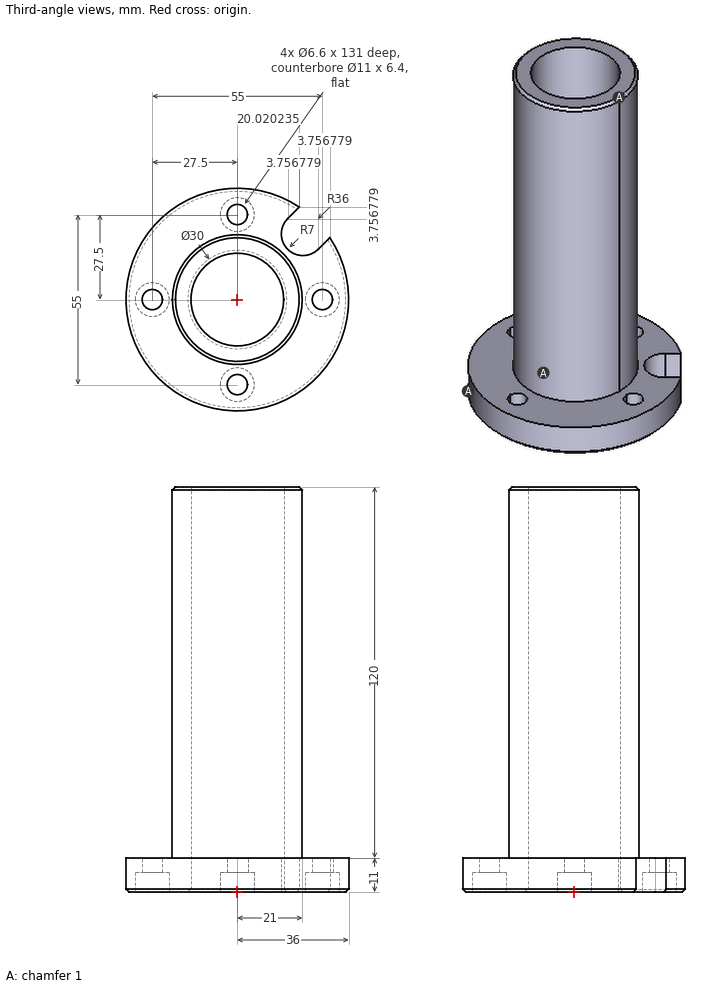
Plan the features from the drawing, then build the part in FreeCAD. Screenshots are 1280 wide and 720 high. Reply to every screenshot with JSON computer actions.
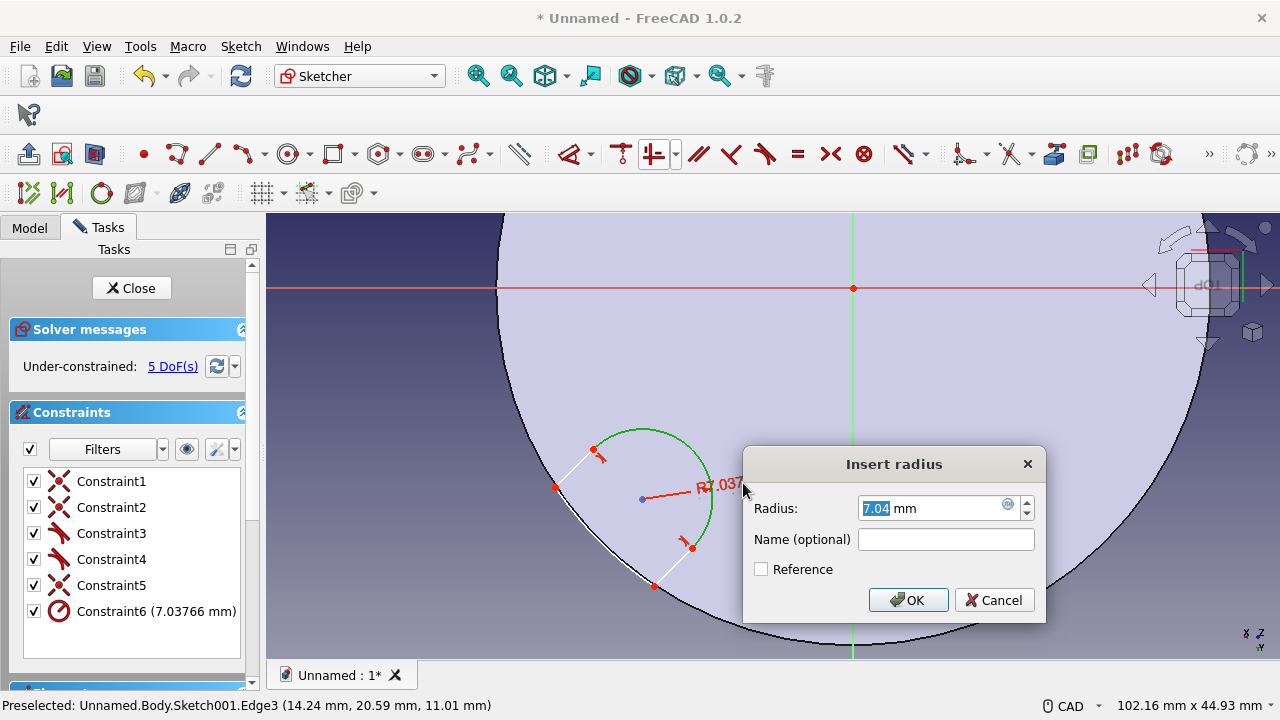
{"action": "type", "text": "7"}
{"action": "key", "text": "Return"}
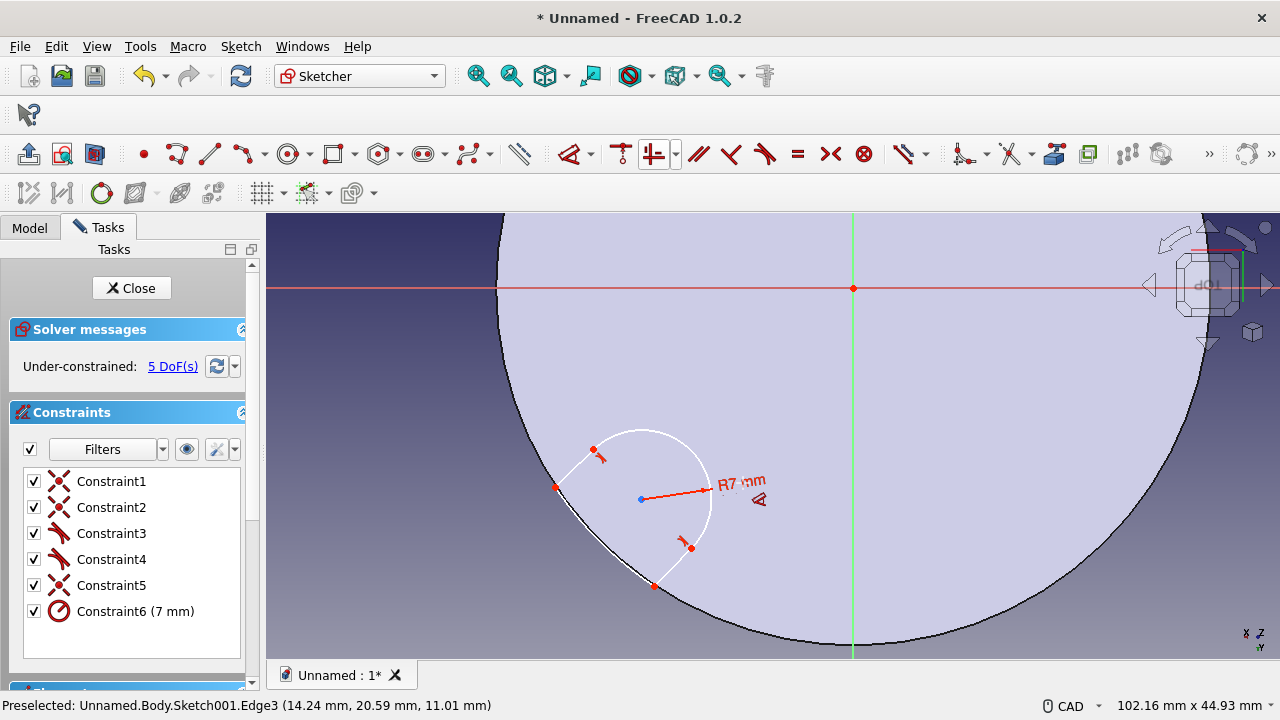
{"action": "left_click", "coordinate": [581, 521]}
{"action": "left_click", "coordinate": [557, 542]}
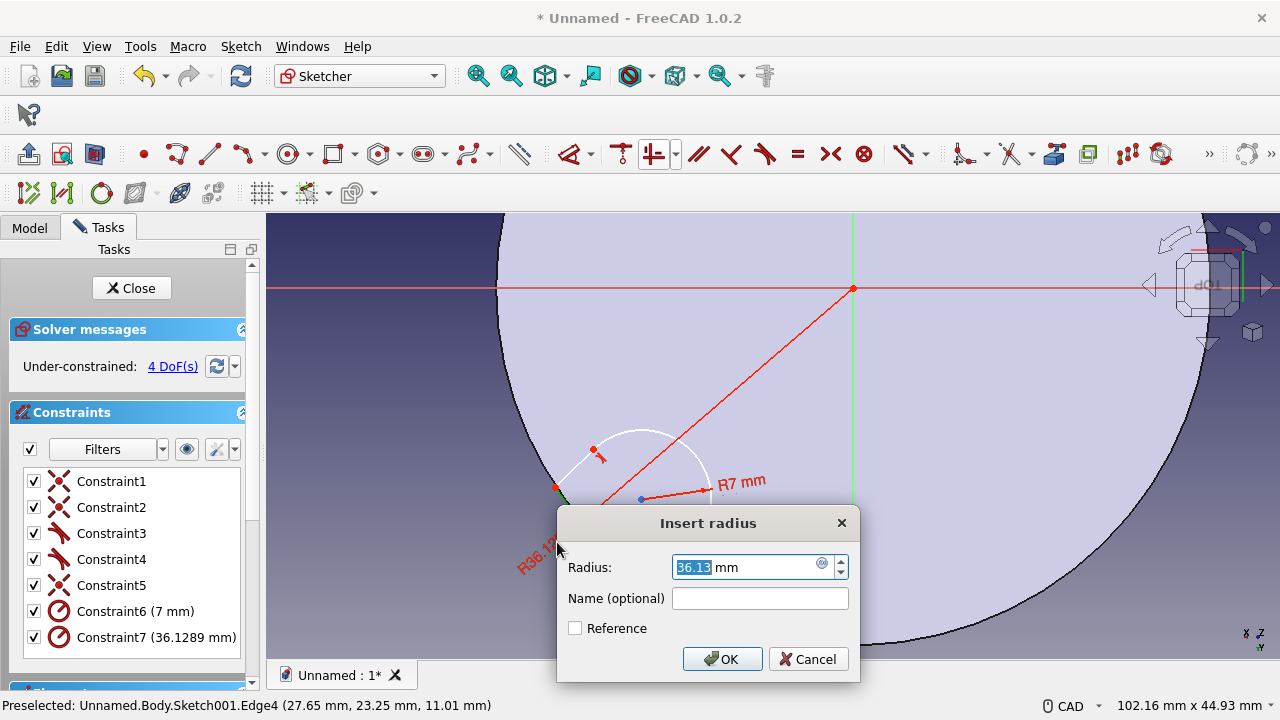
{"action": "type", "text": "36"}
{"action": "key", "text": "Return"}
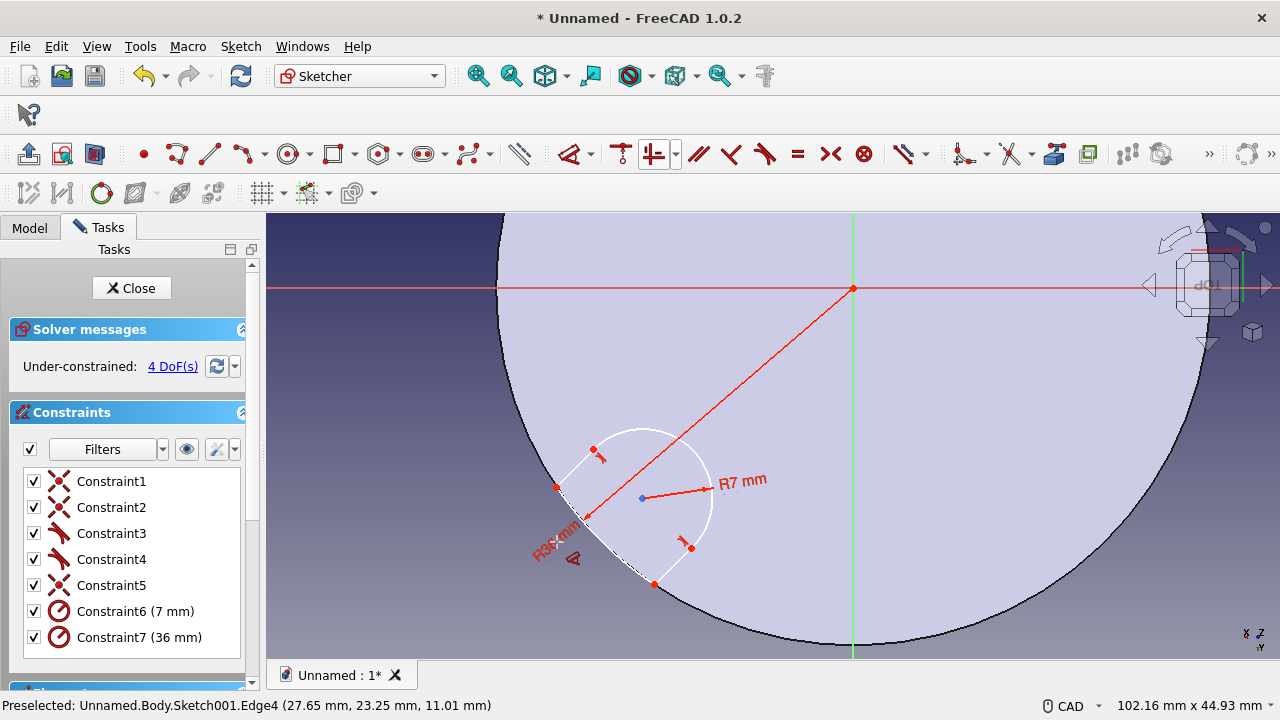
{"action": "left_click", "coordinate": [665, 574]}
{"action": "left_click", "coordinate": [673, 619]}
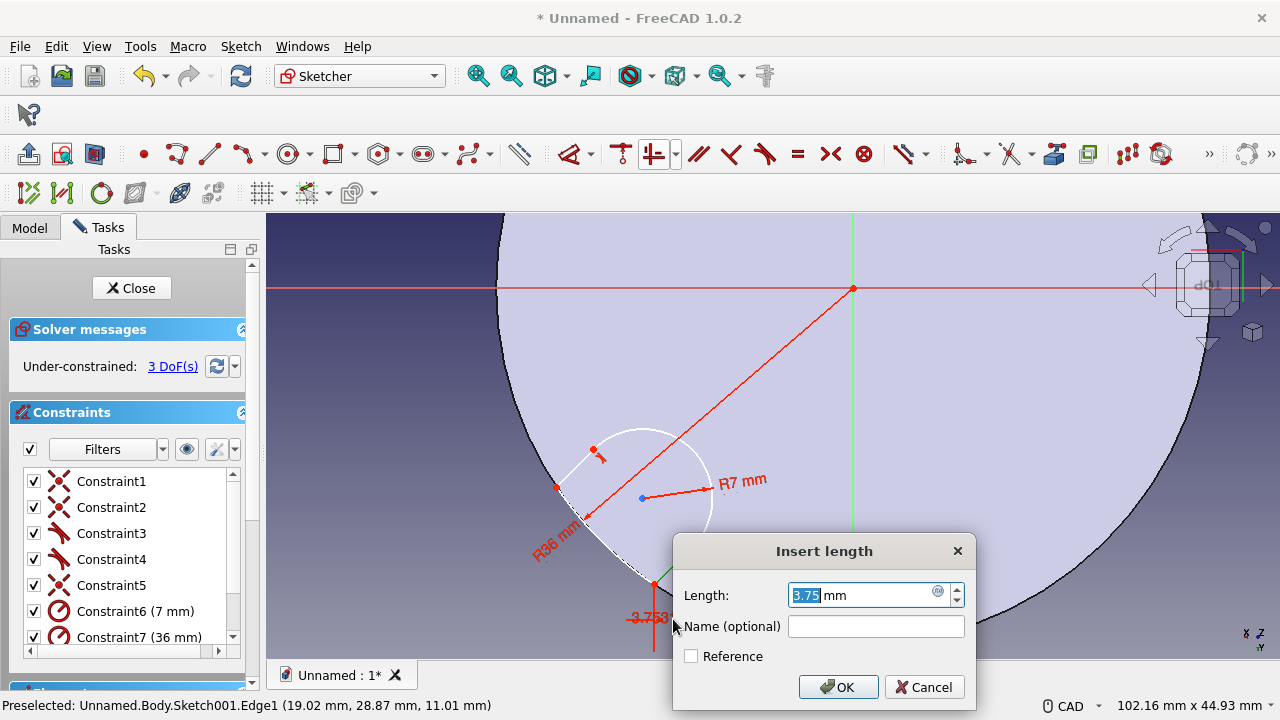
{"action": "type", "text": "3.756779"}
{"action": "key", "text": "Return"}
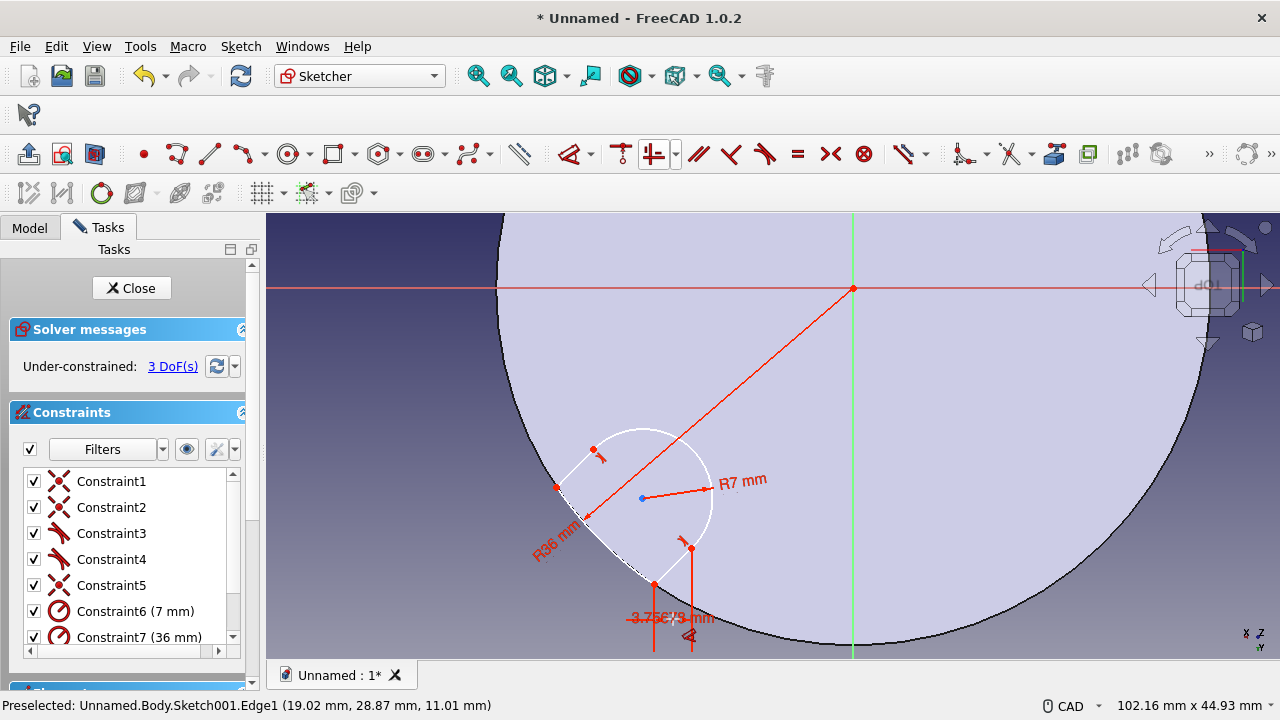
{"action": "left_click", "coordinate": [665, 574]}
{"action": "left_click", "coordinate": [620, 579]}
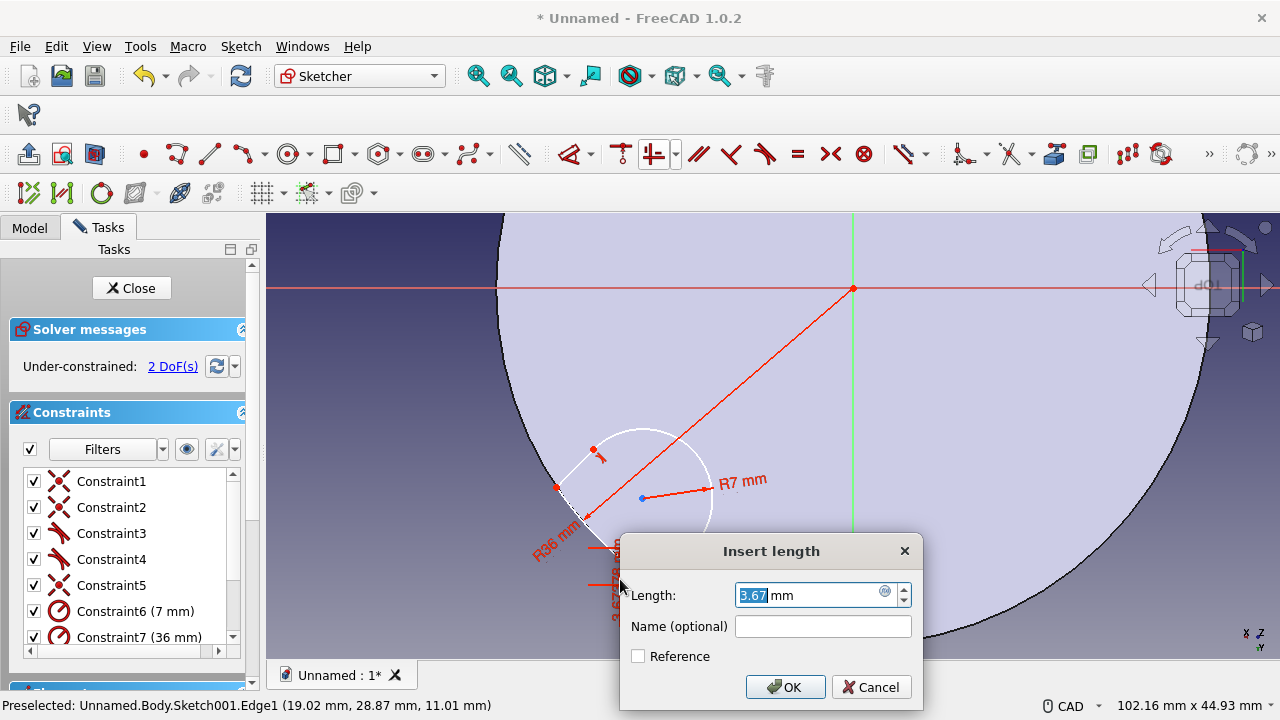
{"action": "type", "text": "3.756779"}
{"action": "key", "text": "Return"}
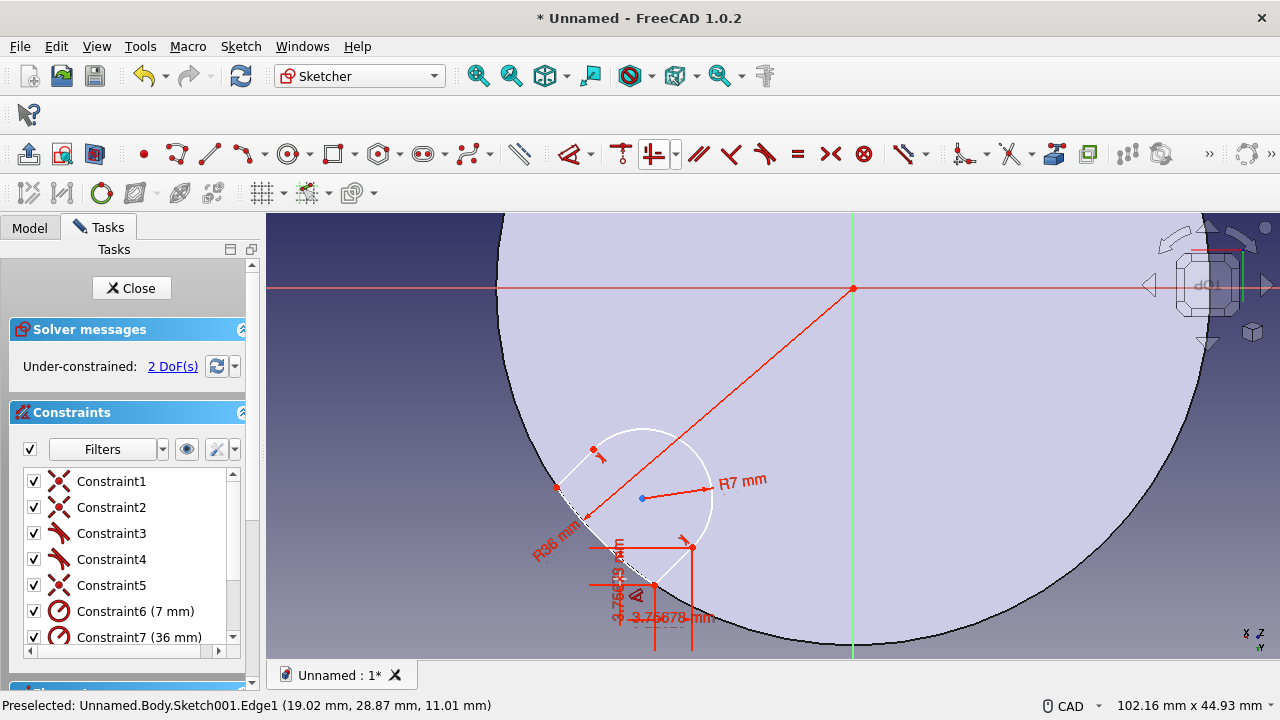
{"action": "left_click", "coordinate": [582, 461]}
{"action": "left_click", "coordinate": [562, 521]}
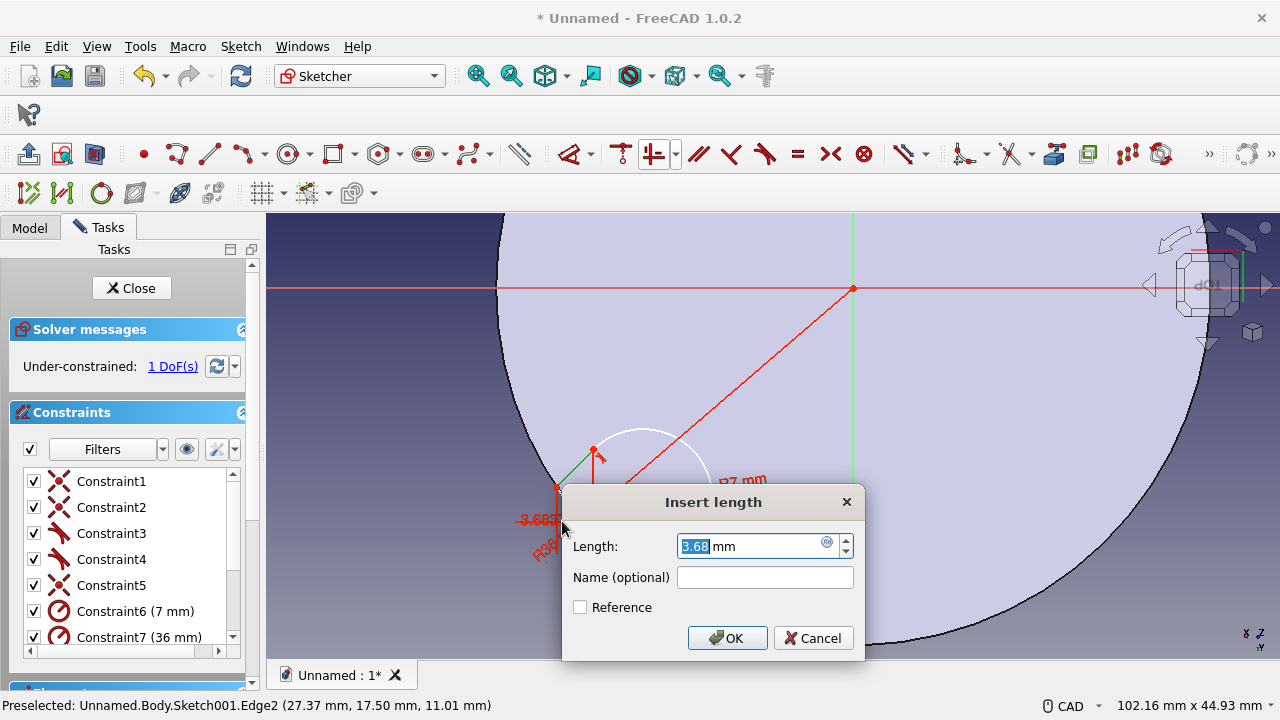
{"action": "type", "text": "3.756779"}
{"action": "key", "text": "Return"}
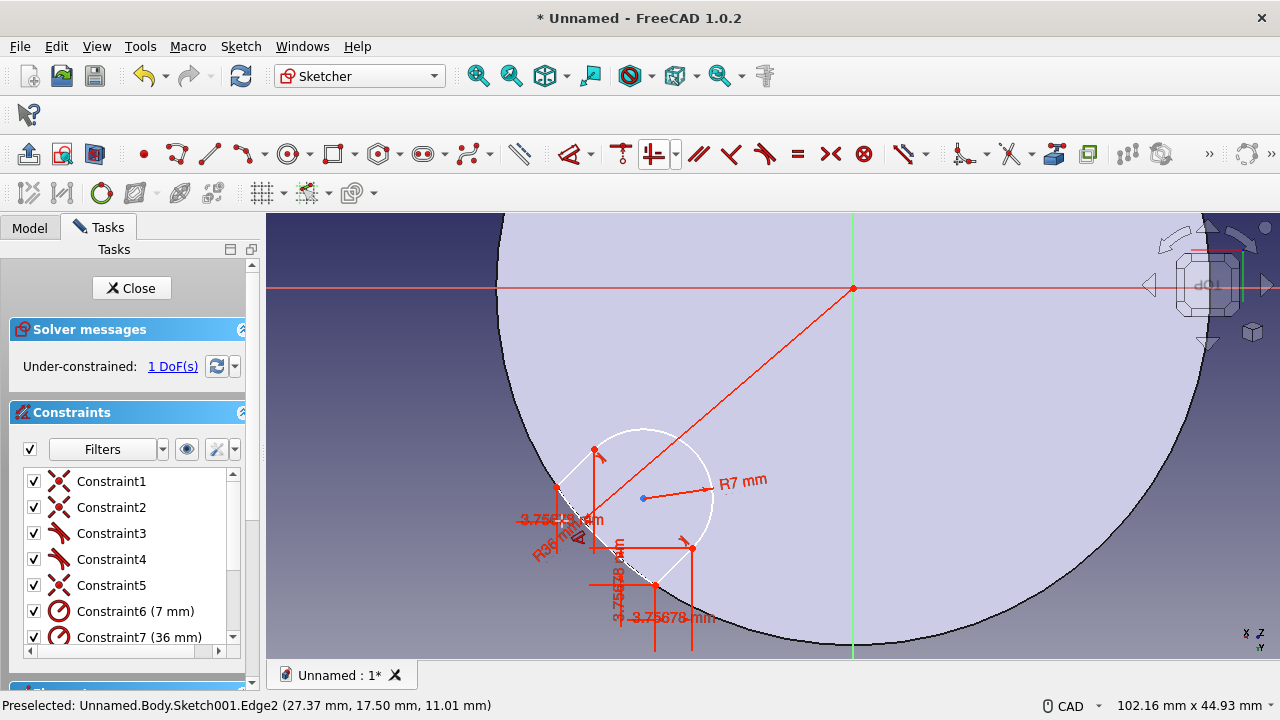
{"action": "left_click", "coordinate": [655, 585]}
{"action": "left_click", "coordinate": [754, 619]}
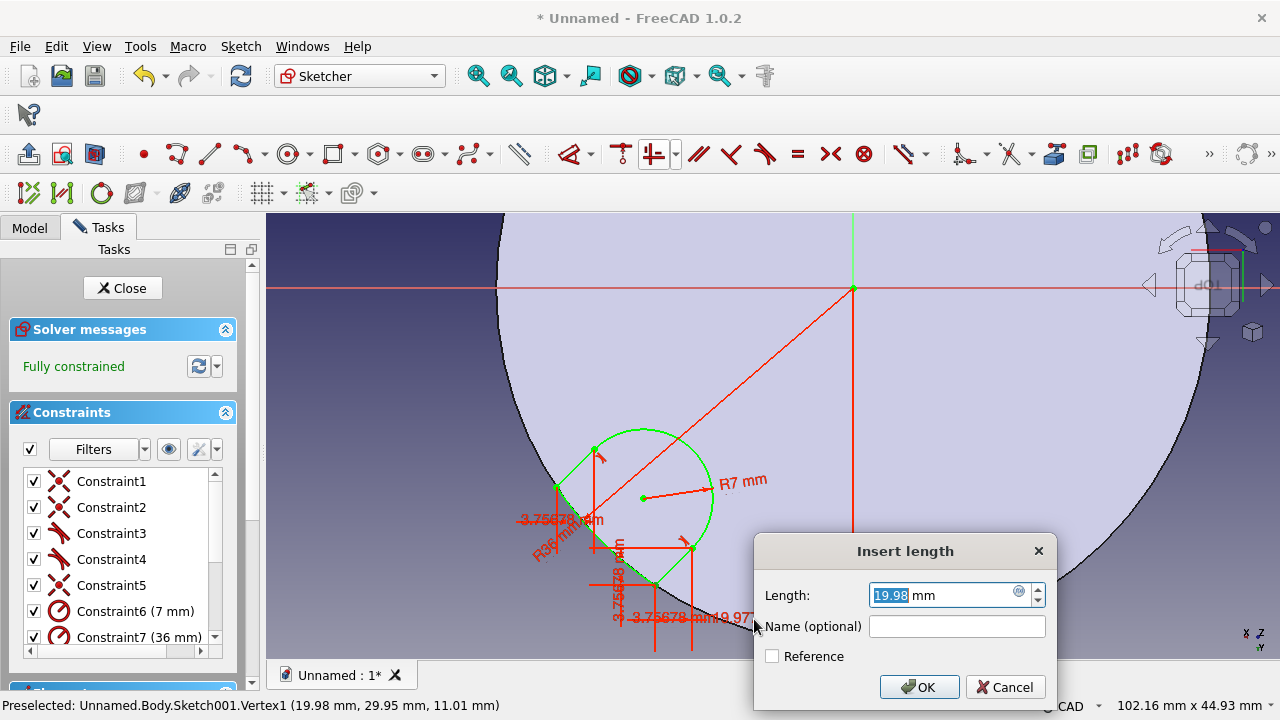
{"action": "type", "text": "20.020235"}
{"action": "key", "text": "Return"}
{"action": "key", "text": "Escape"}